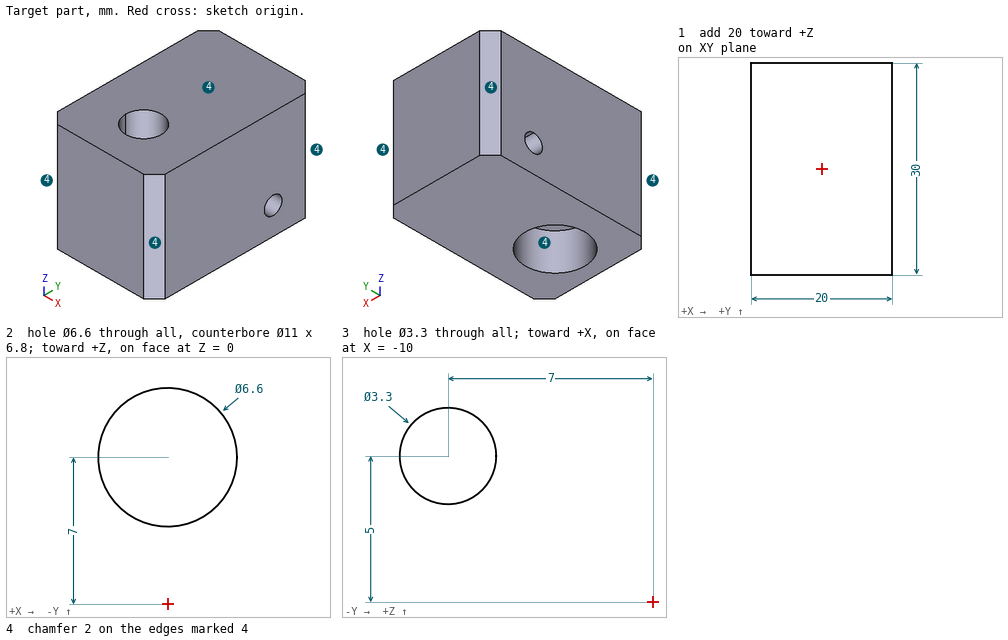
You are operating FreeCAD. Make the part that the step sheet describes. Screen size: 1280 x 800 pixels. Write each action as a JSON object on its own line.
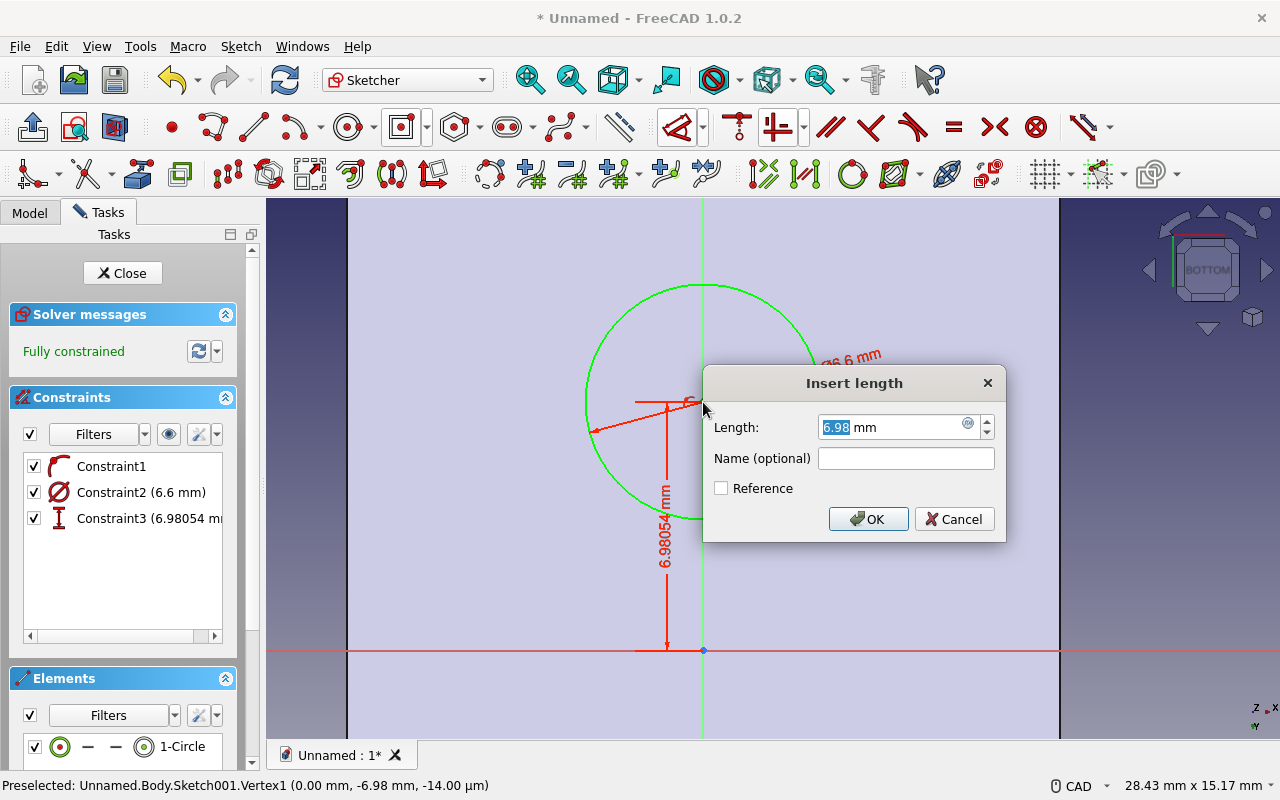
{"action": "type", "text": "7"}
{"action": "key", "text": "Return"}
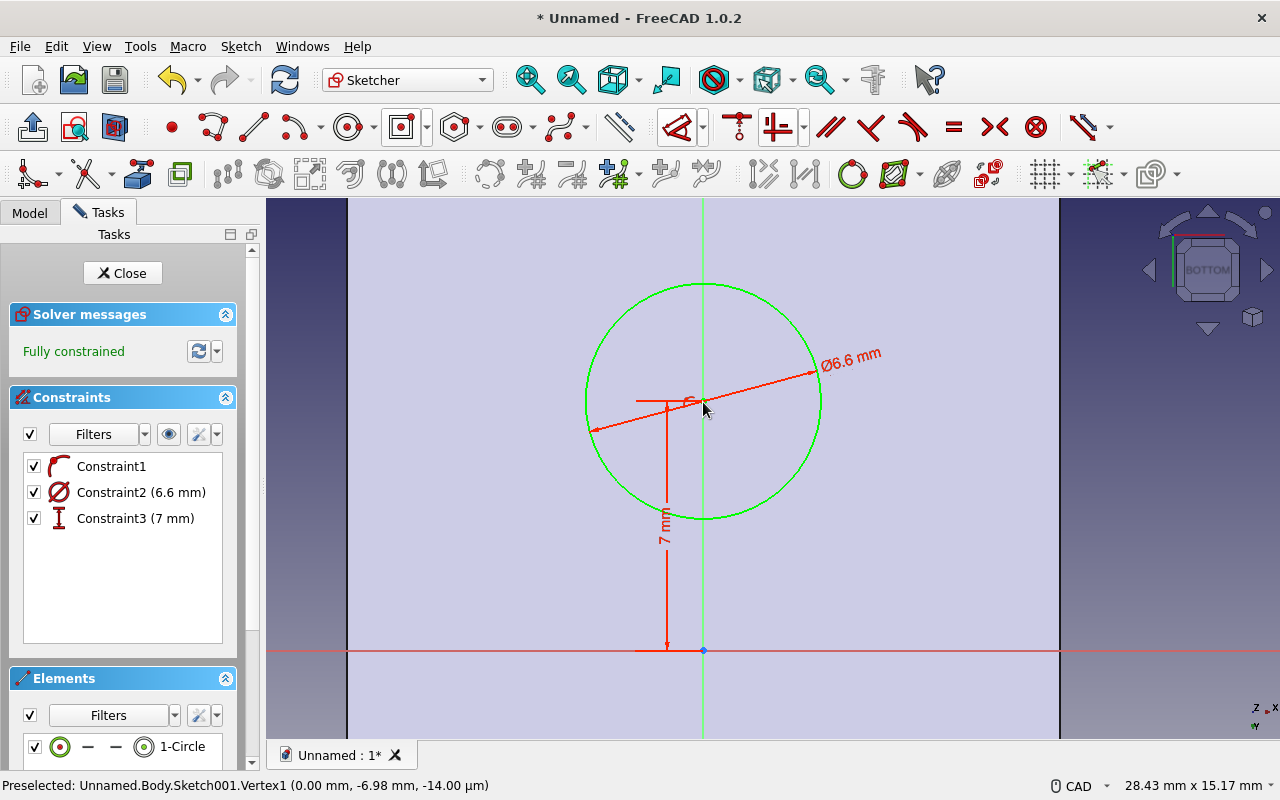
{"action": "left_click", "coordinate": [123, 273]}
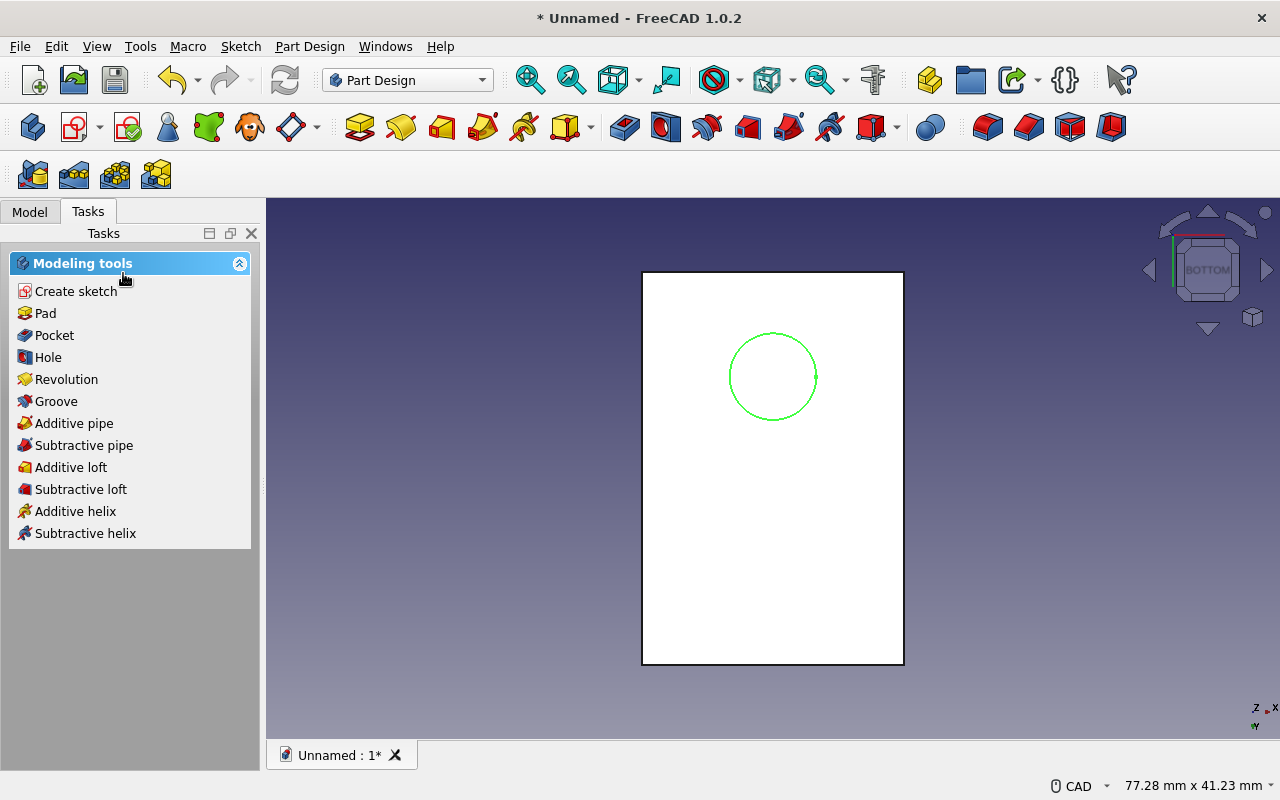
{"action": "left_click", "coordinate": [666, 128]}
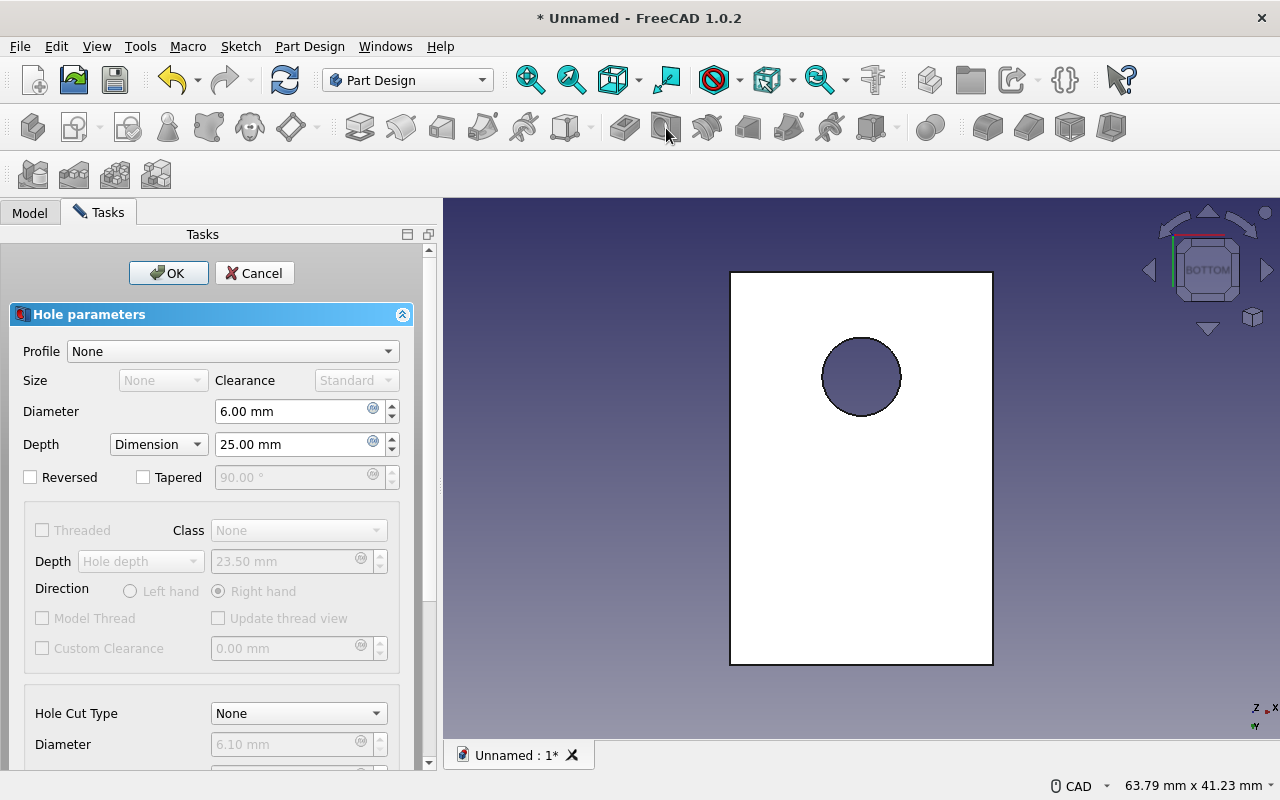
{"action": "triple_click", "coordinate": [300, 412]}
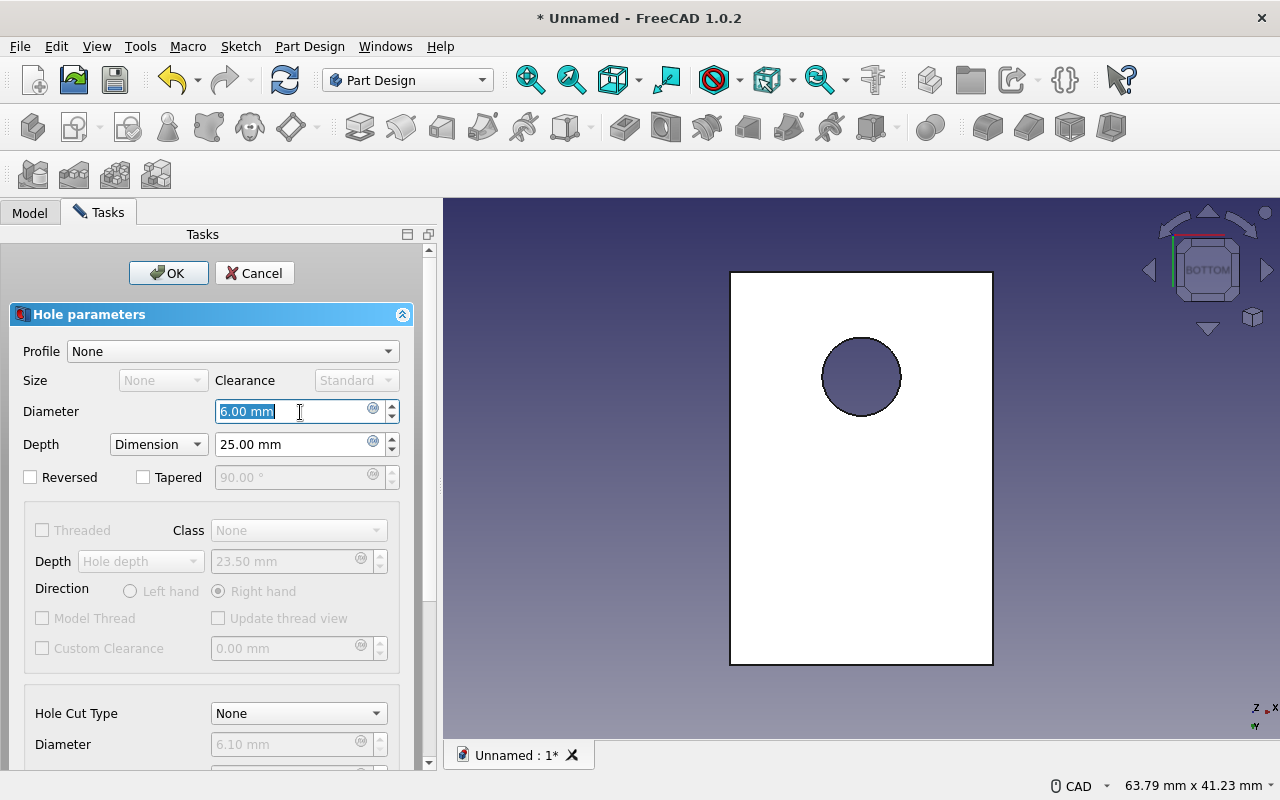
{"action": "type", "text": "6.6"}
{"action": "key", "text": "Tab"}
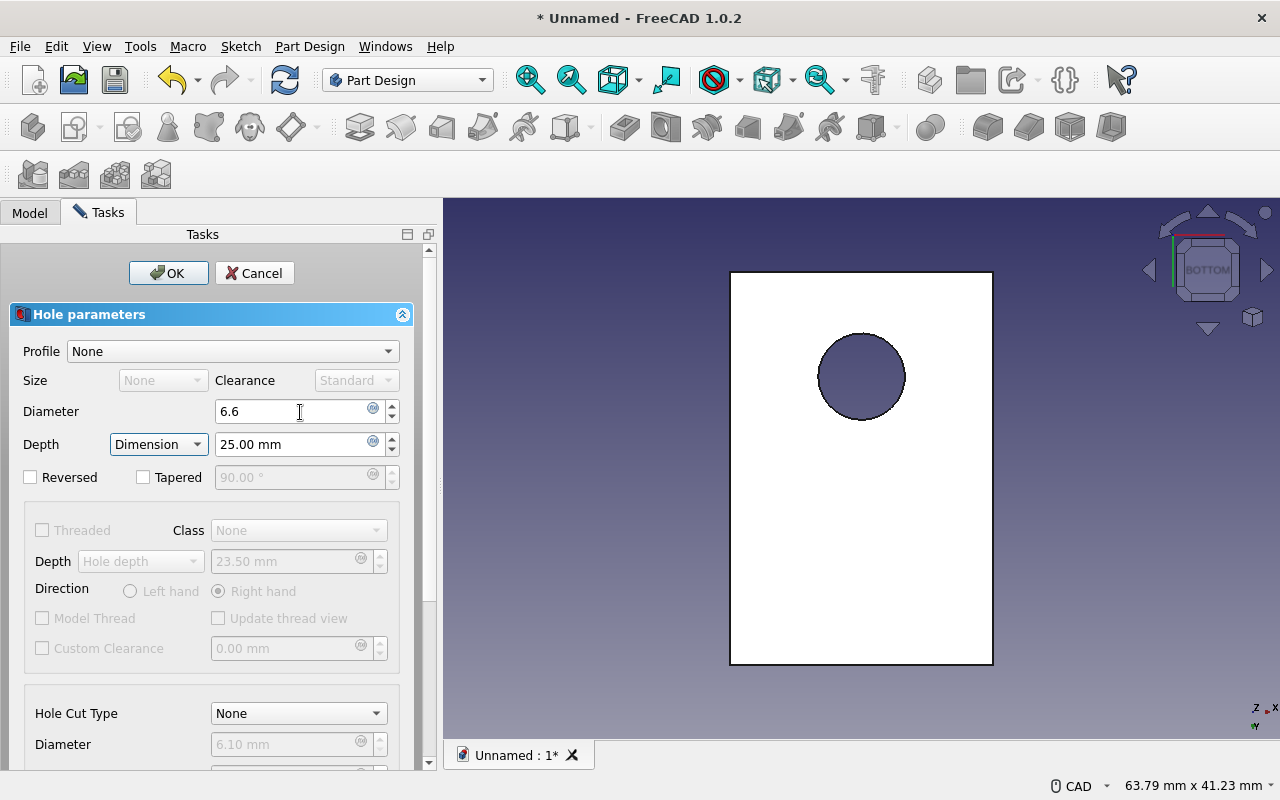
{"action": "left_click", "coordinate": [160, 444]}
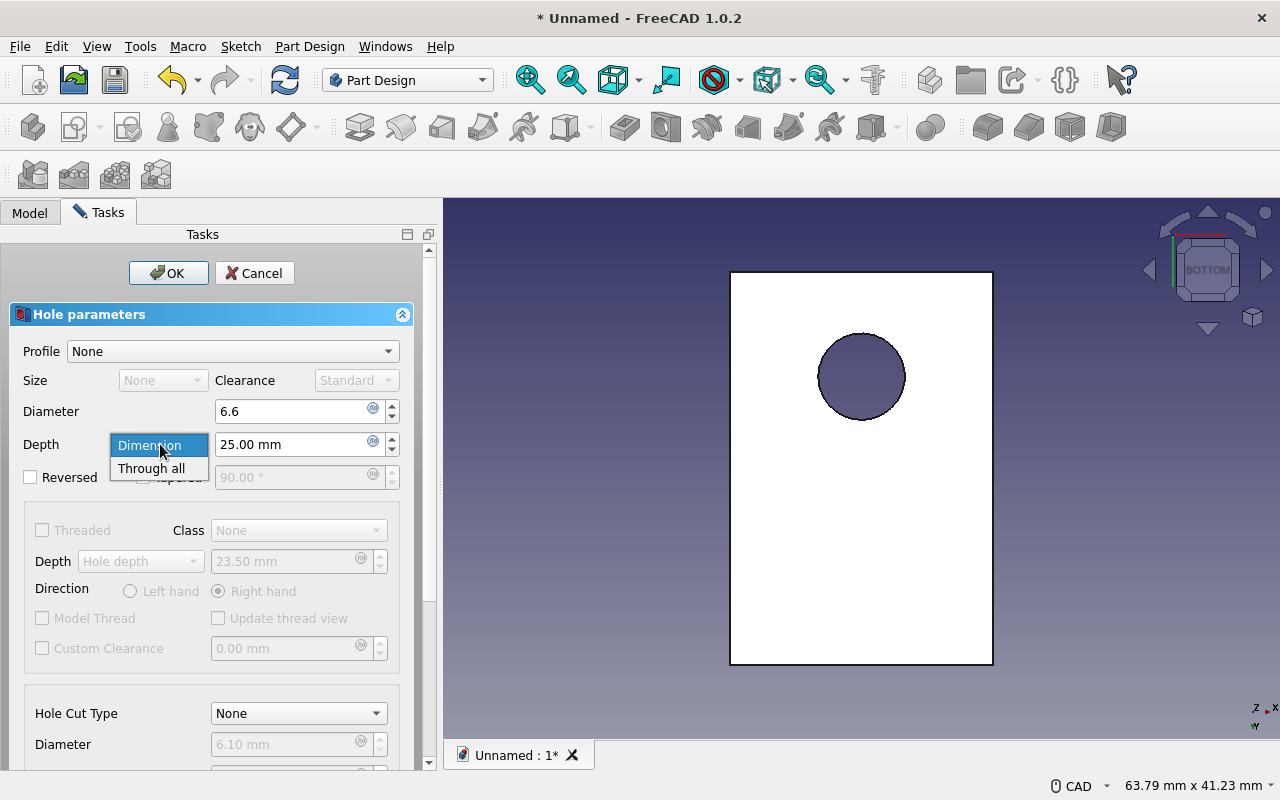
{"action": "left_click", "coordinate": [158, 468]}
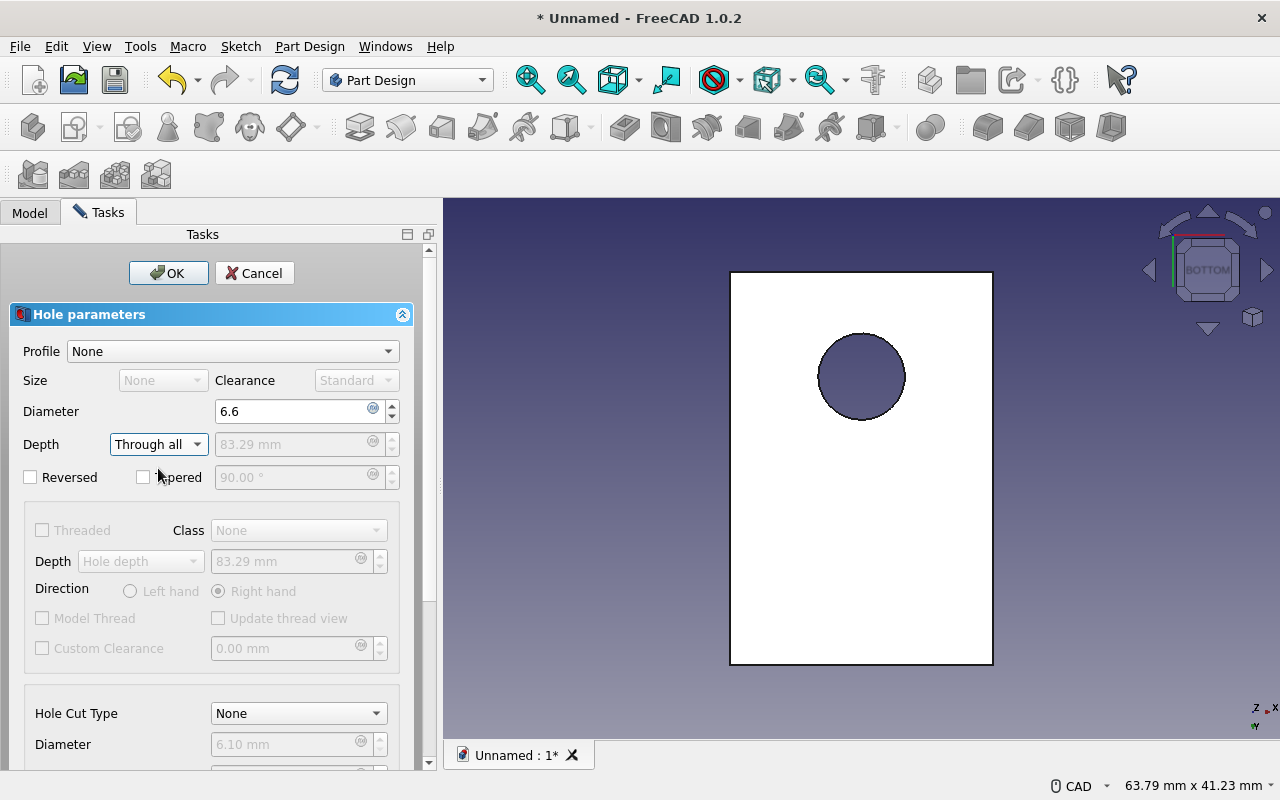
{"action": "left_click", "coordinate": [300, 714]}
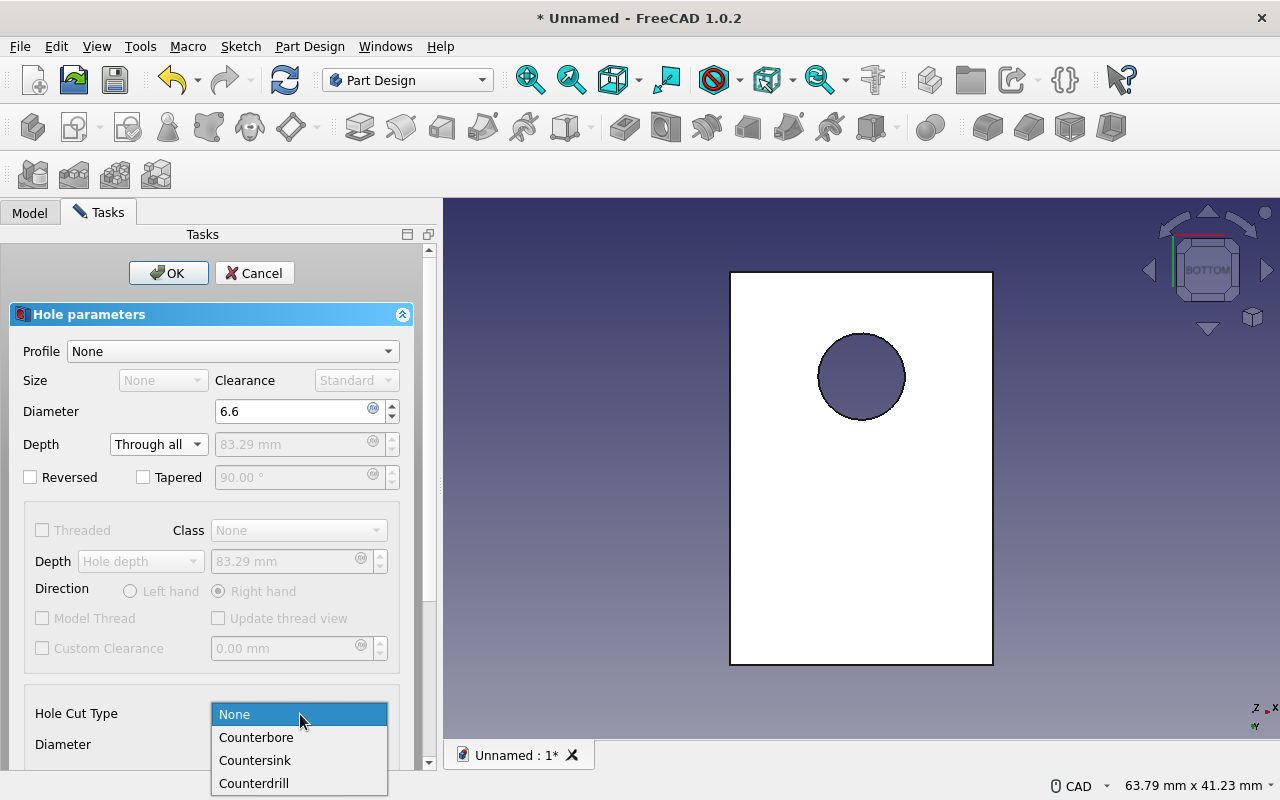
{"action": "left_click", "coordinate": [298, 738]}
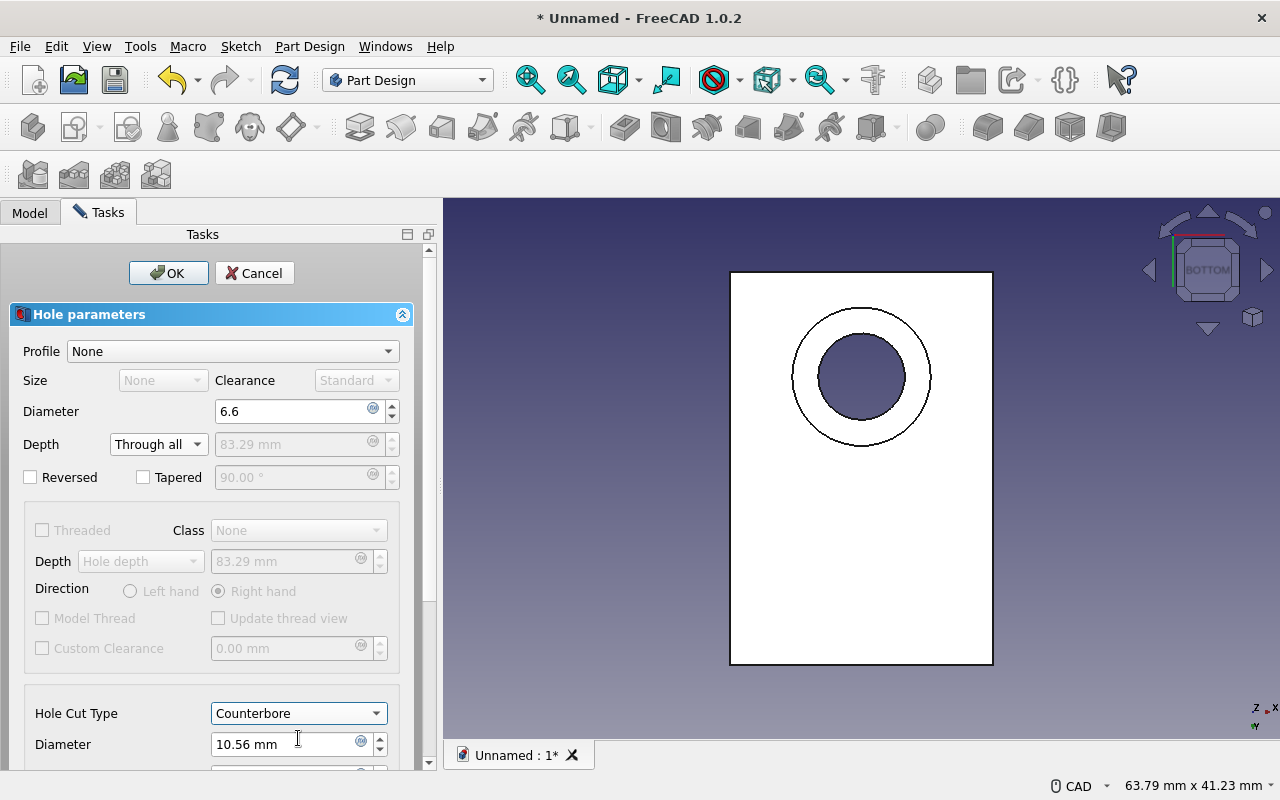
{"action": "triple_click", "coordinate": [292, 744]}